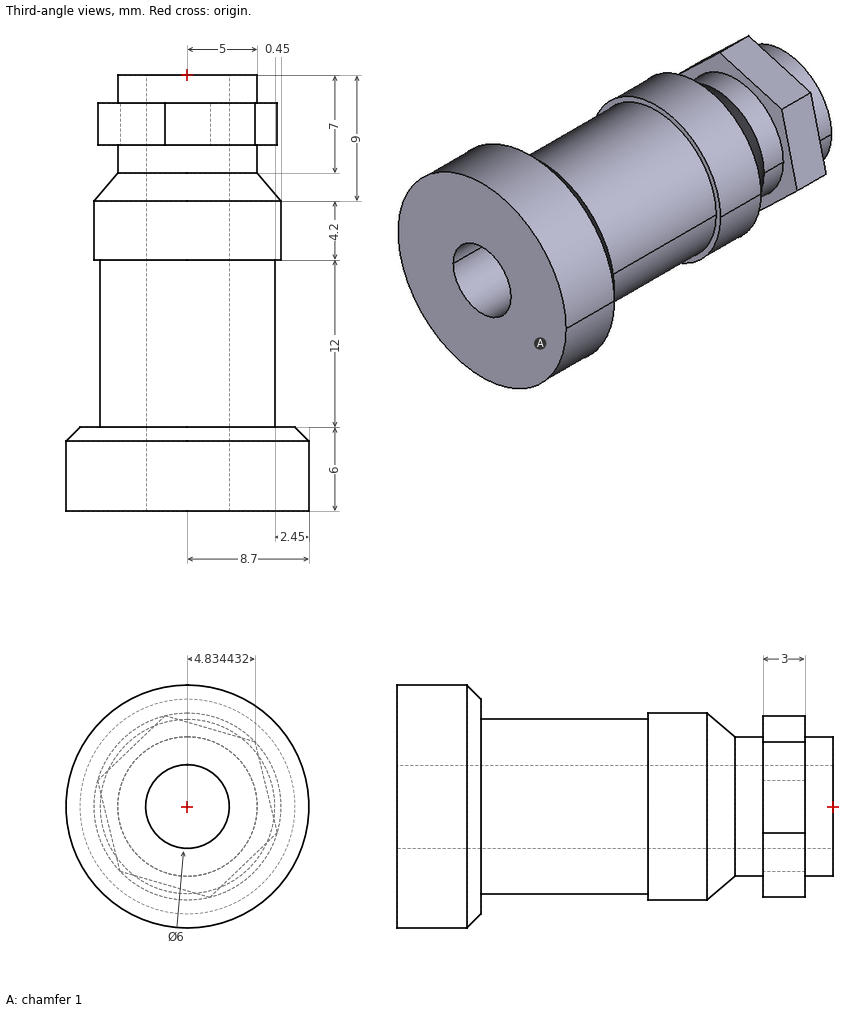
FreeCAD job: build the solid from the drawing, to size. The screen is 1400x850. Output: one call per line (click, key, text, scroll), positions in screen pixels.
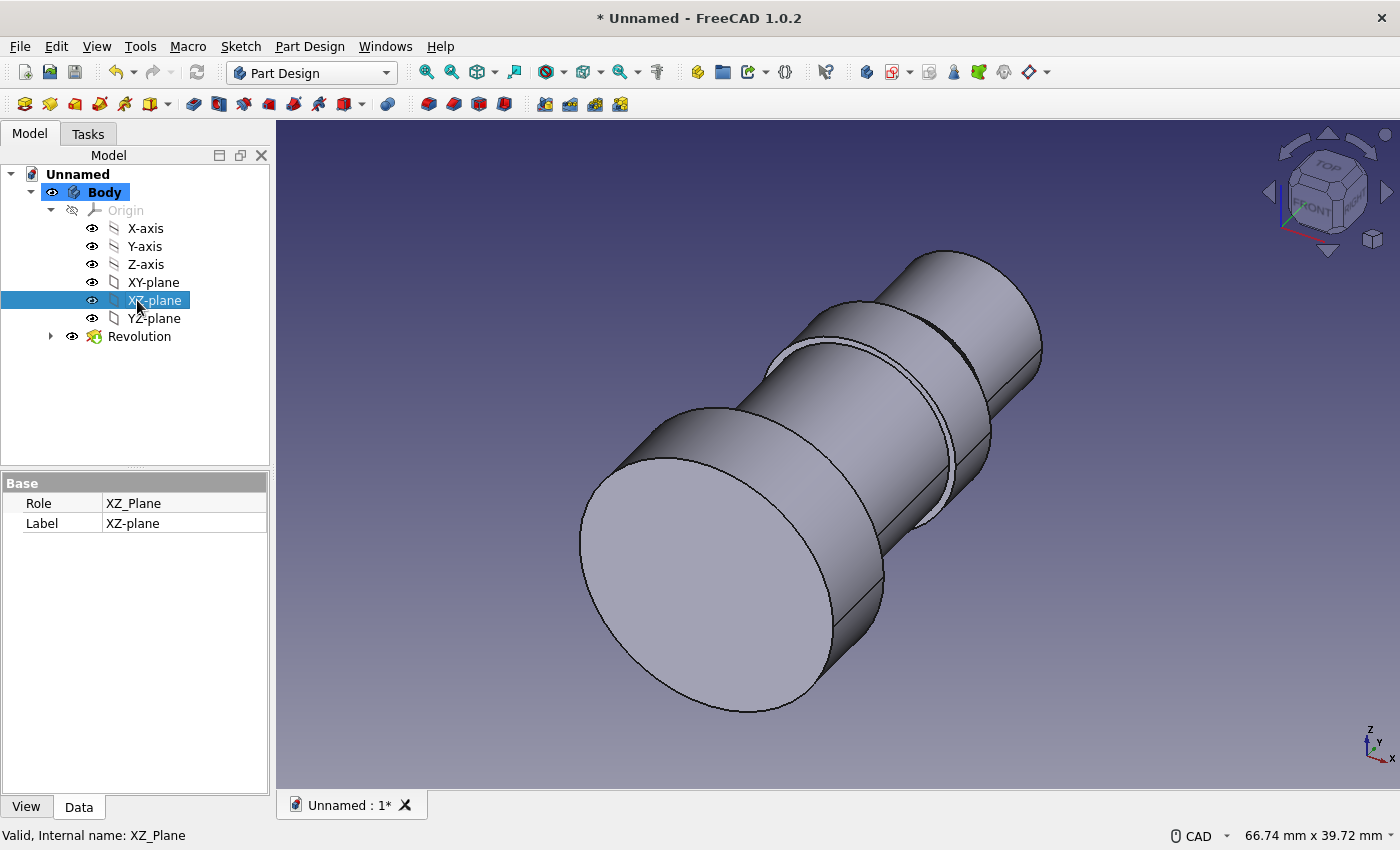
click(1028, 72)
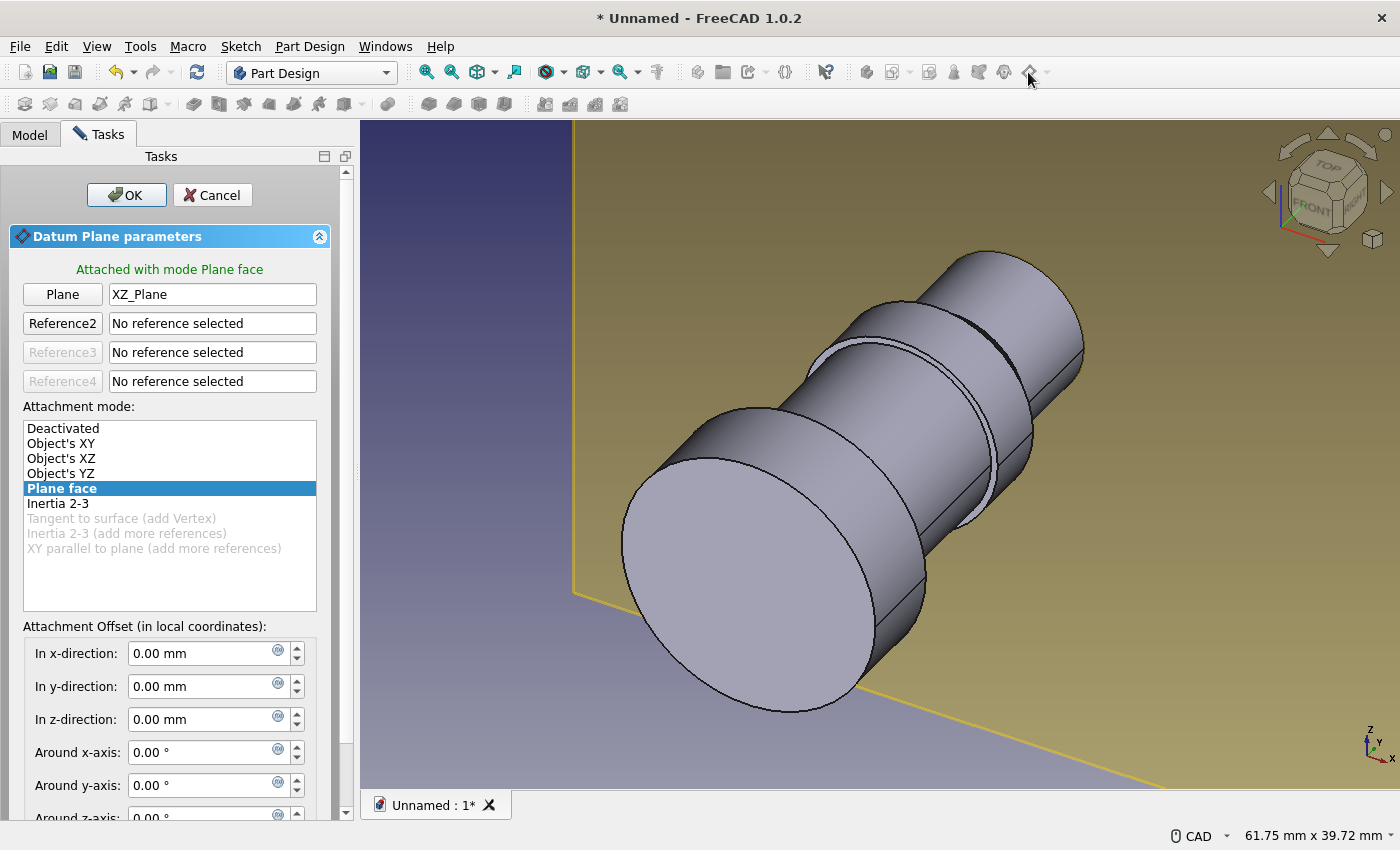
triple_click(210, 720)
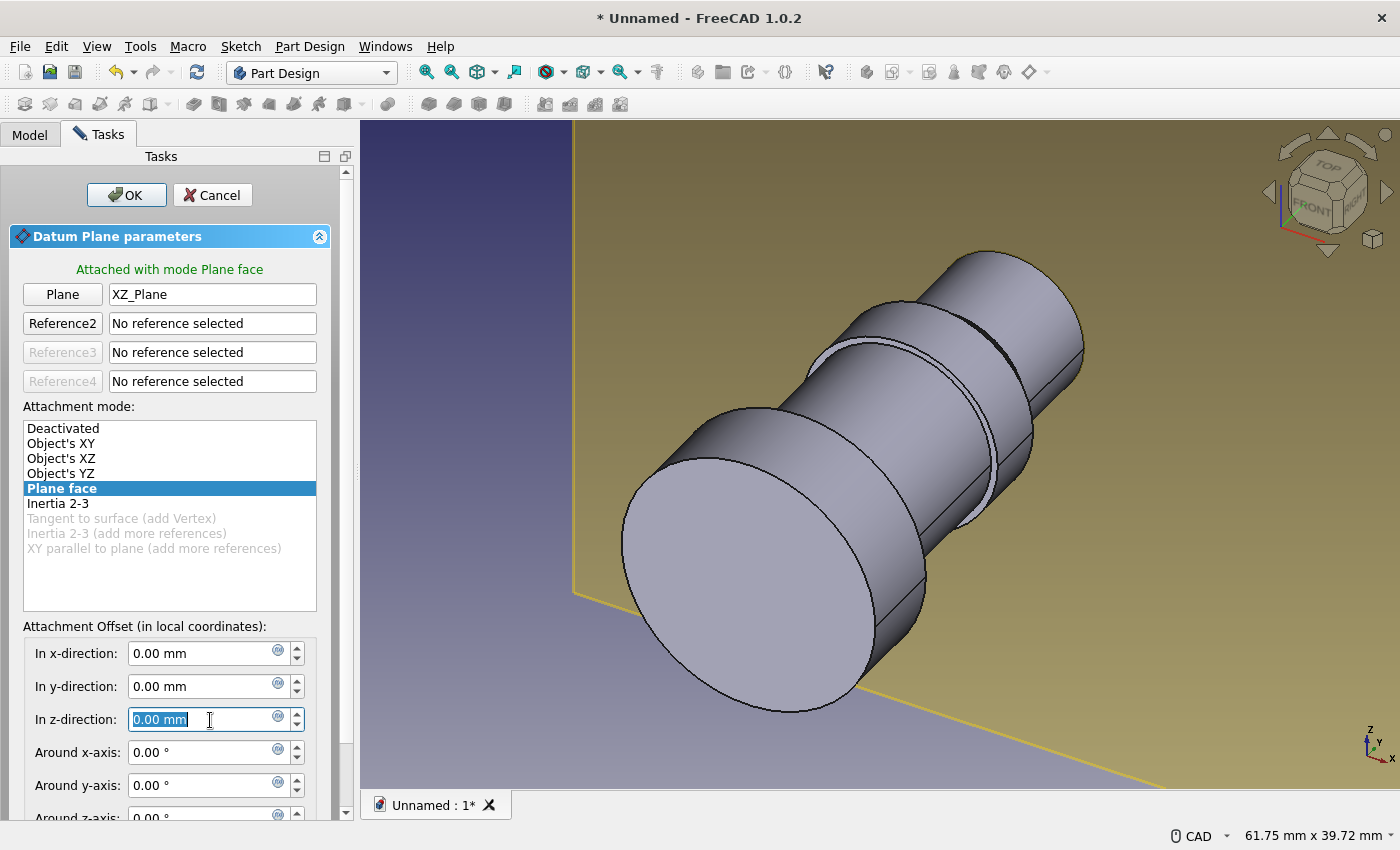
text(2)
key(Tab)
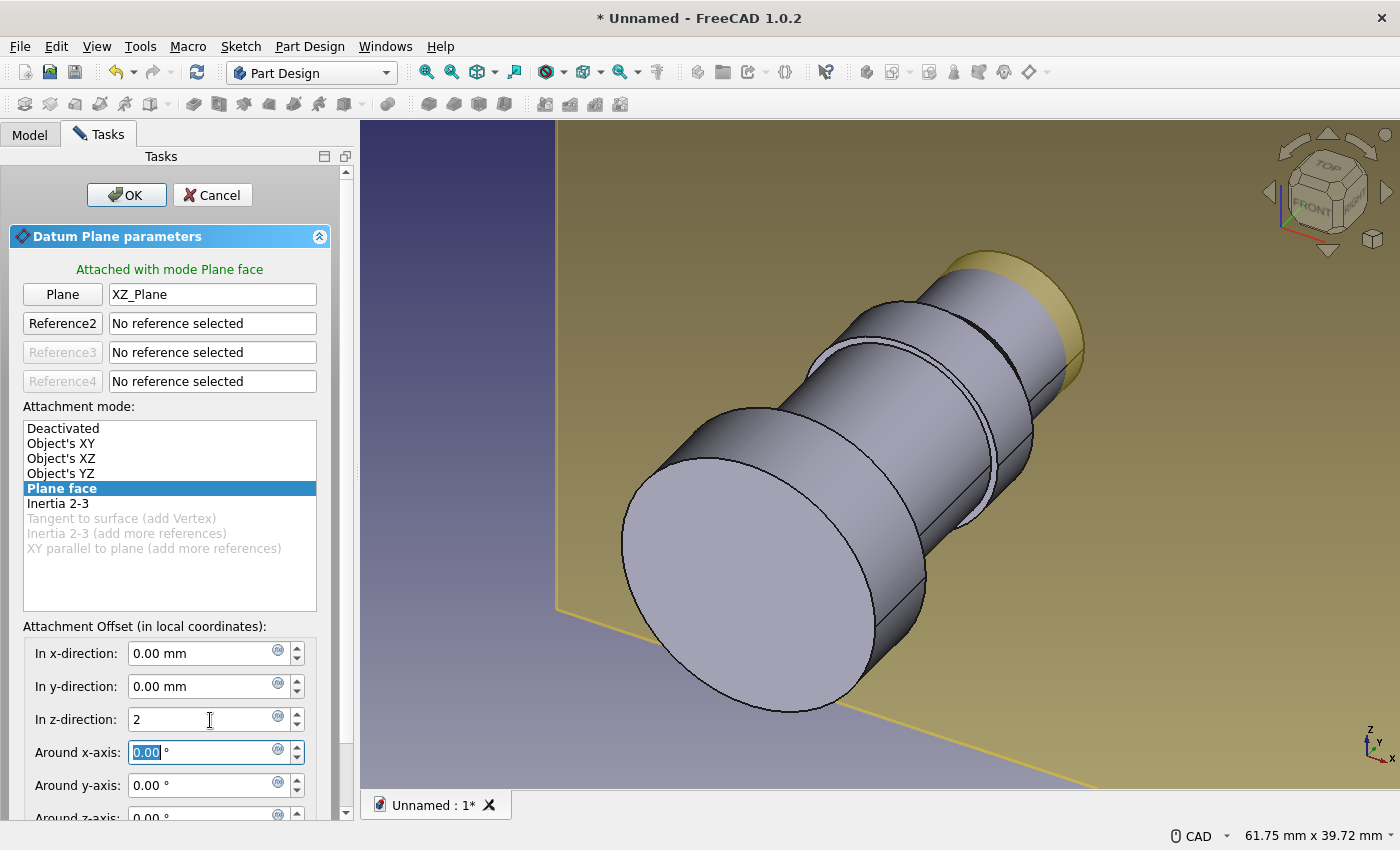
click(127, 195)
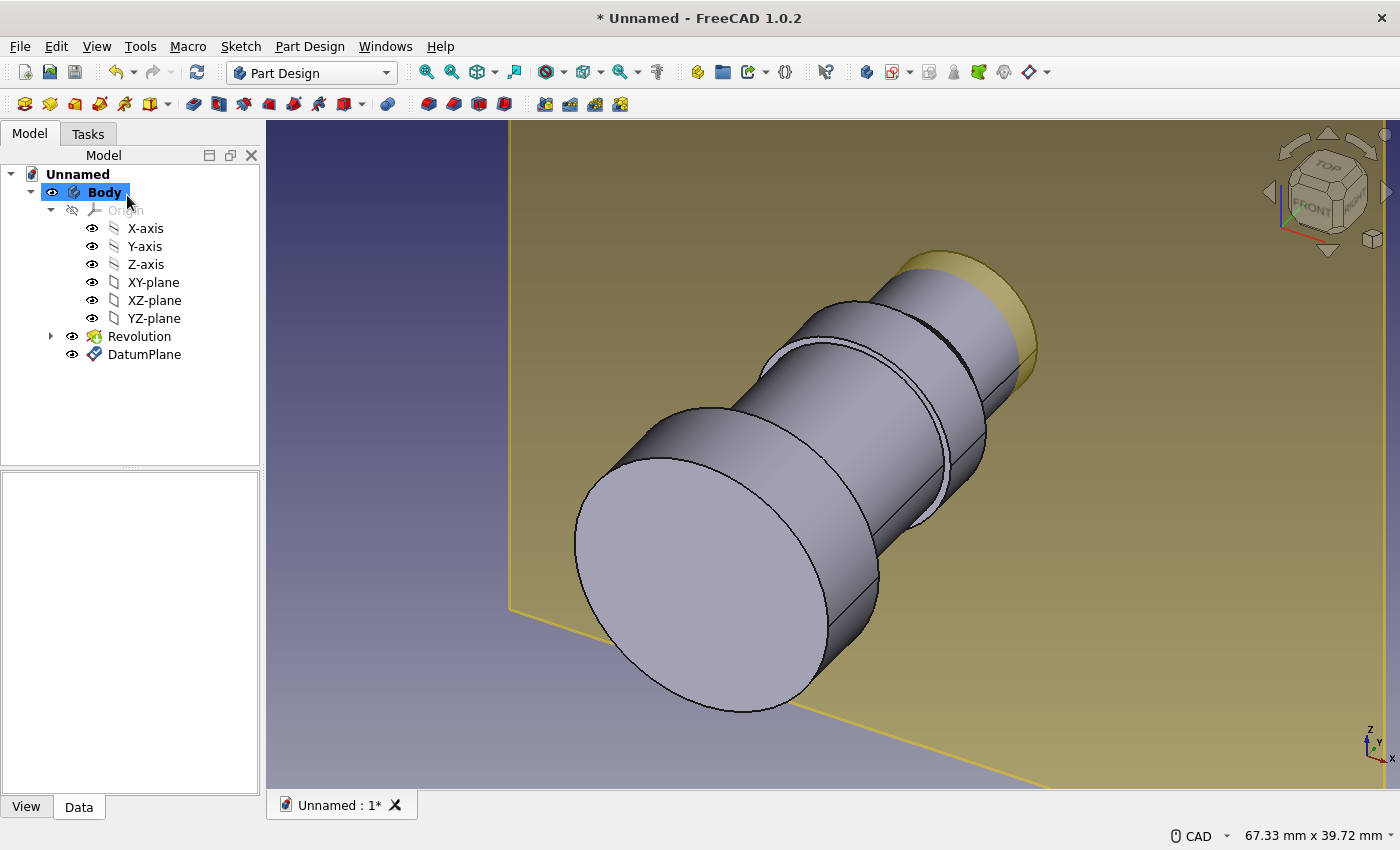
click(117, 354)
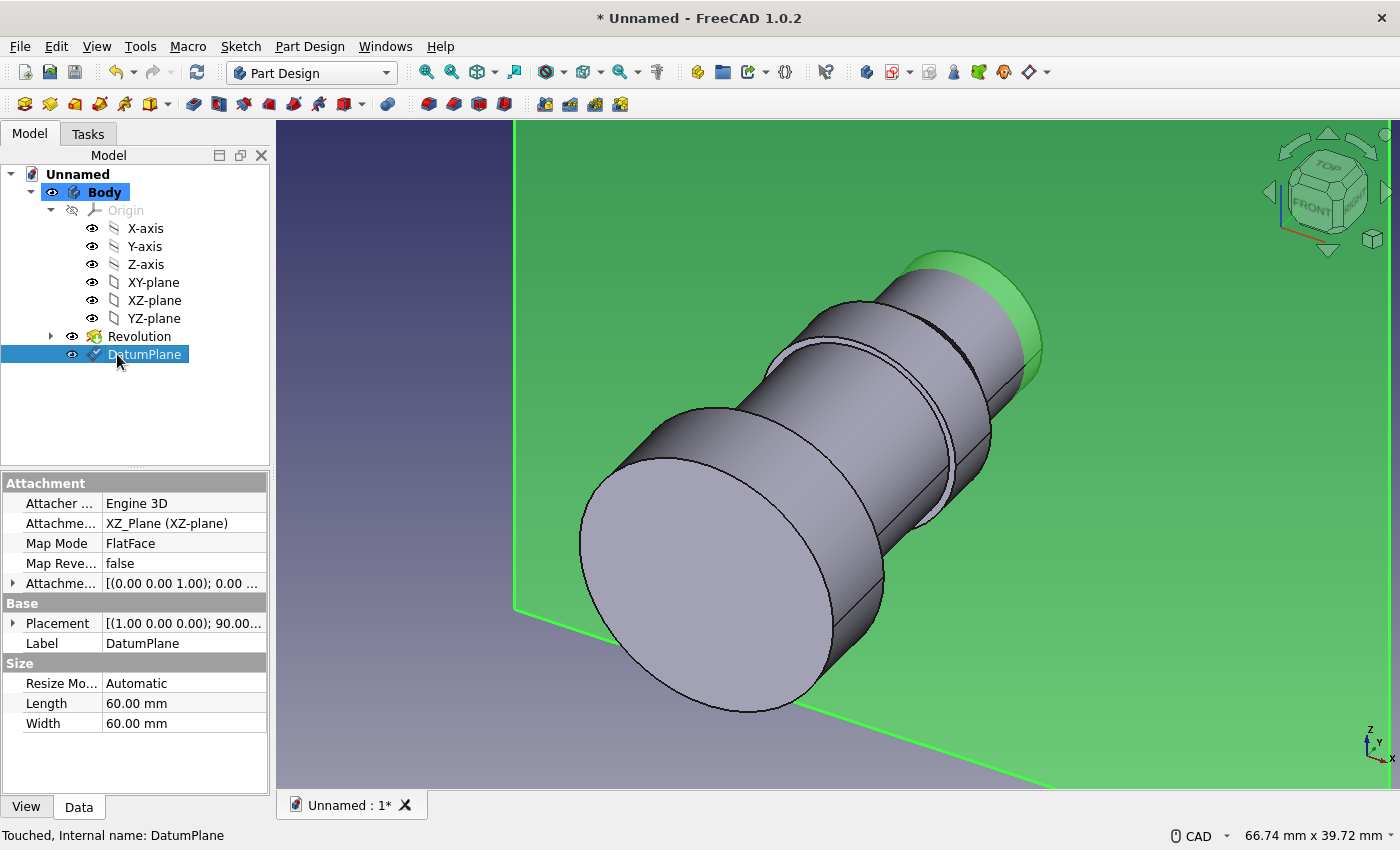
click(892, 72)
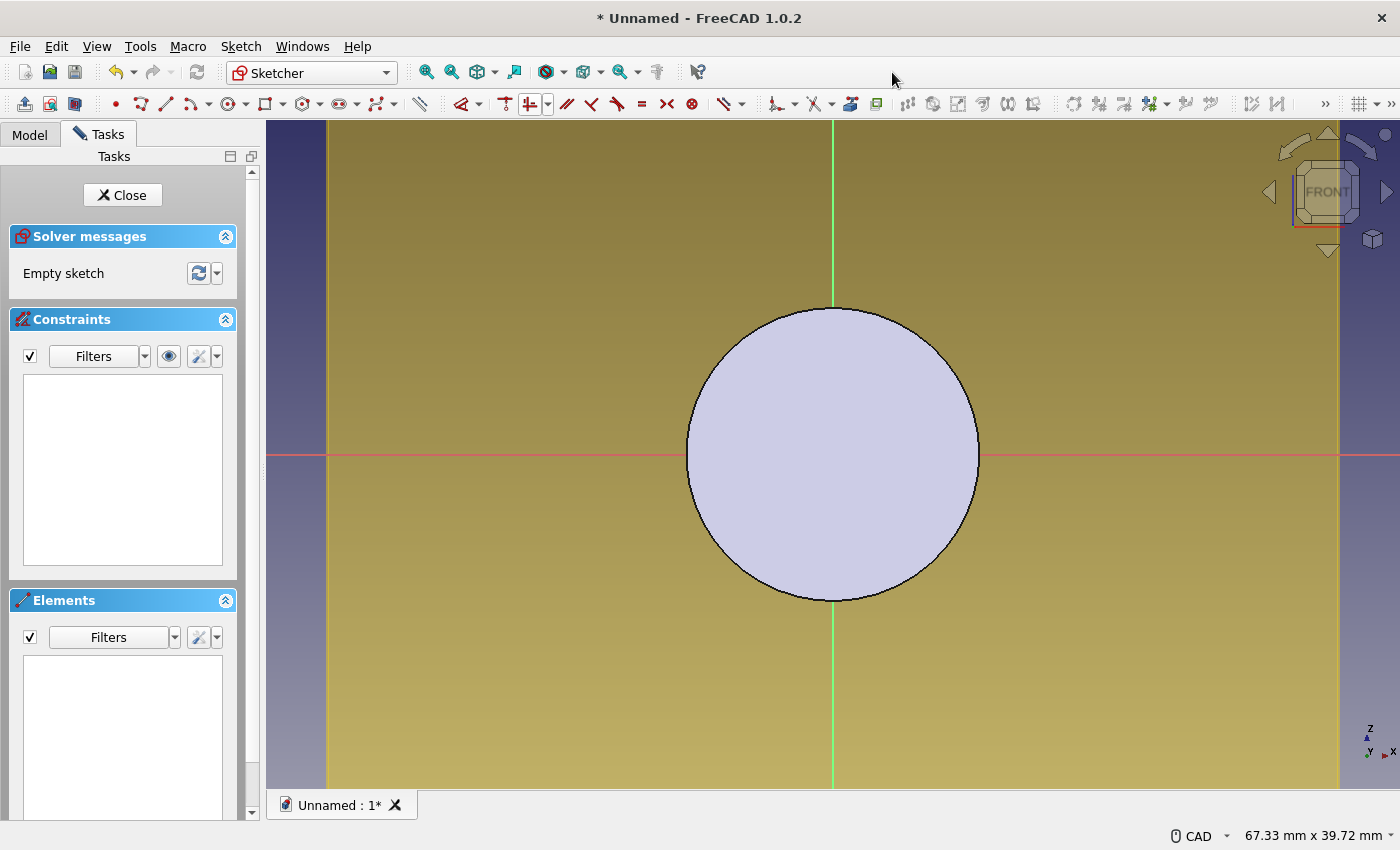
key(q)
key(s)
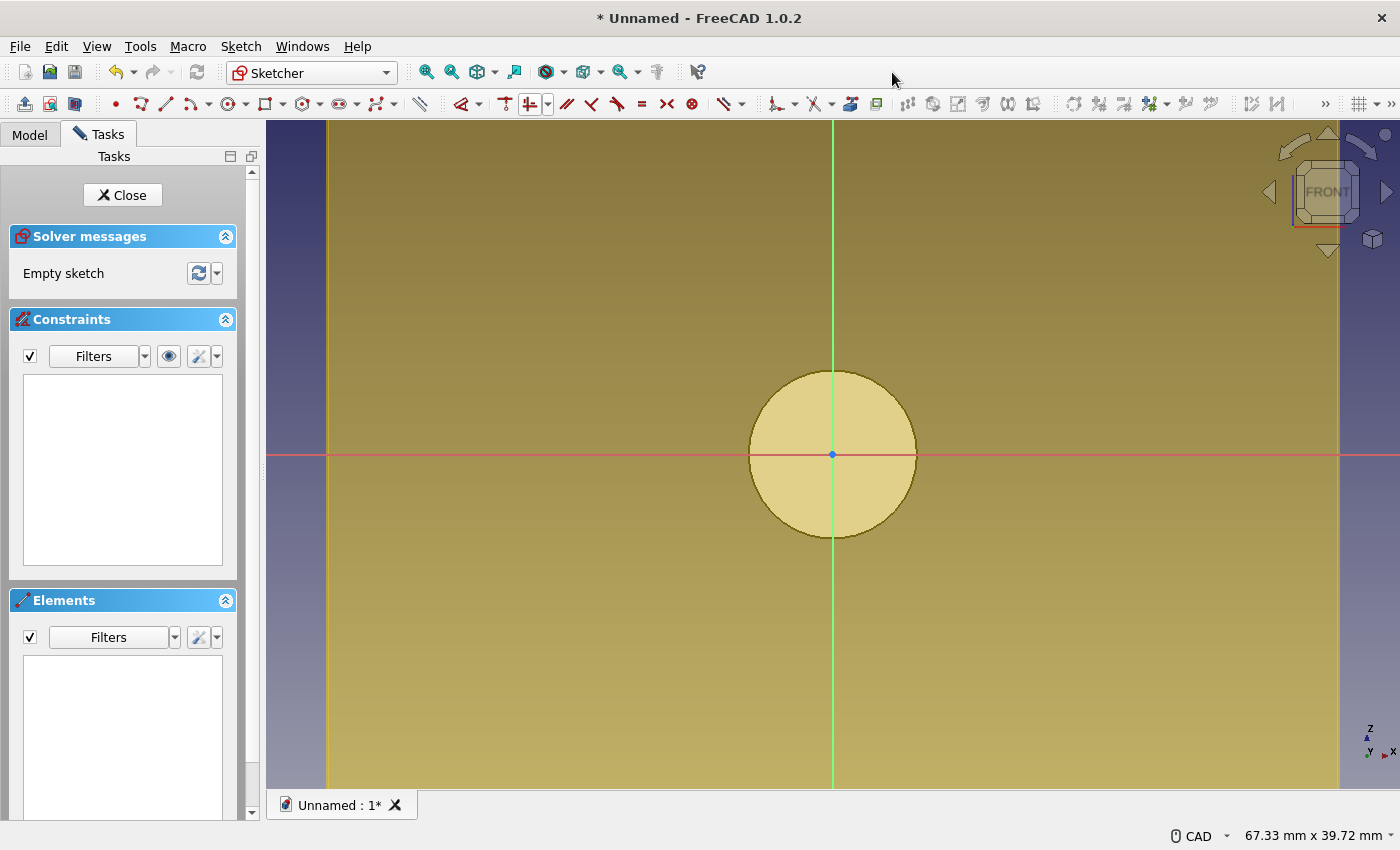
scroll(916, 454, up, 3)